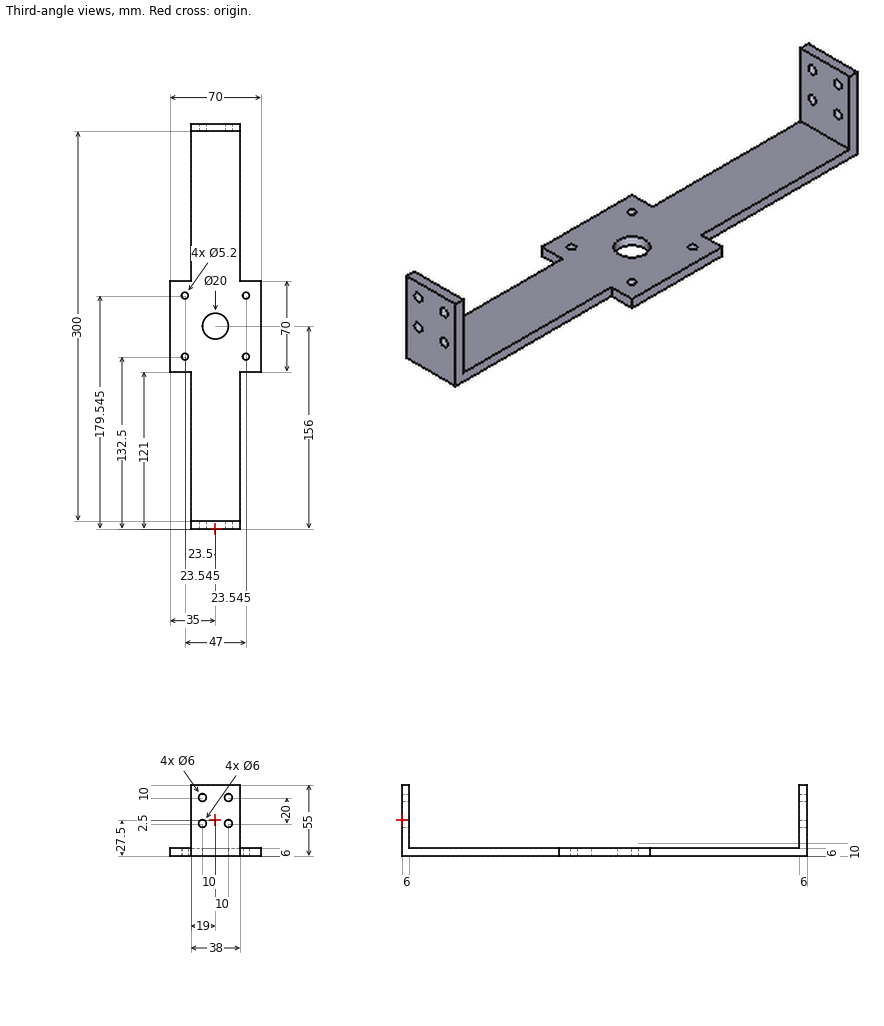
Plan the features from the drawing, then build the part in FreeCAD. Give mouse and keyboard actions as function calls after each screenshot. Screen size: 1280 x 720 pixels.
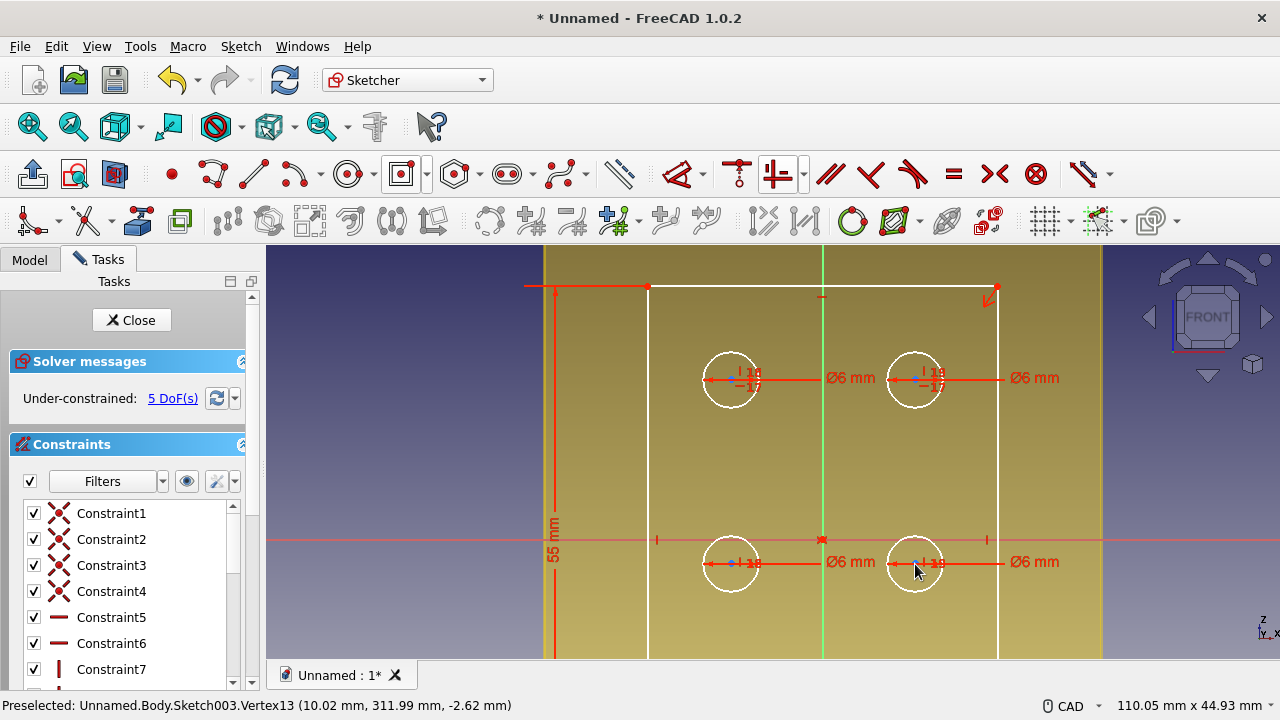
click(731, 564)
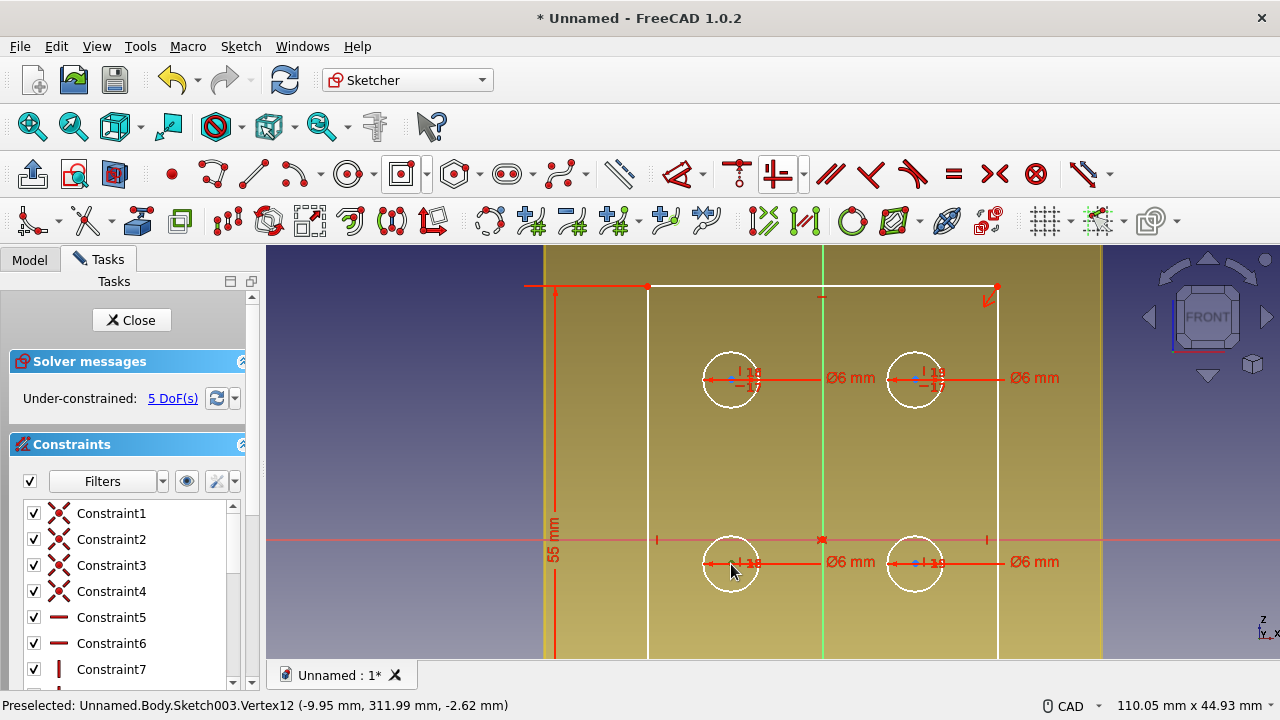
click(915, 564)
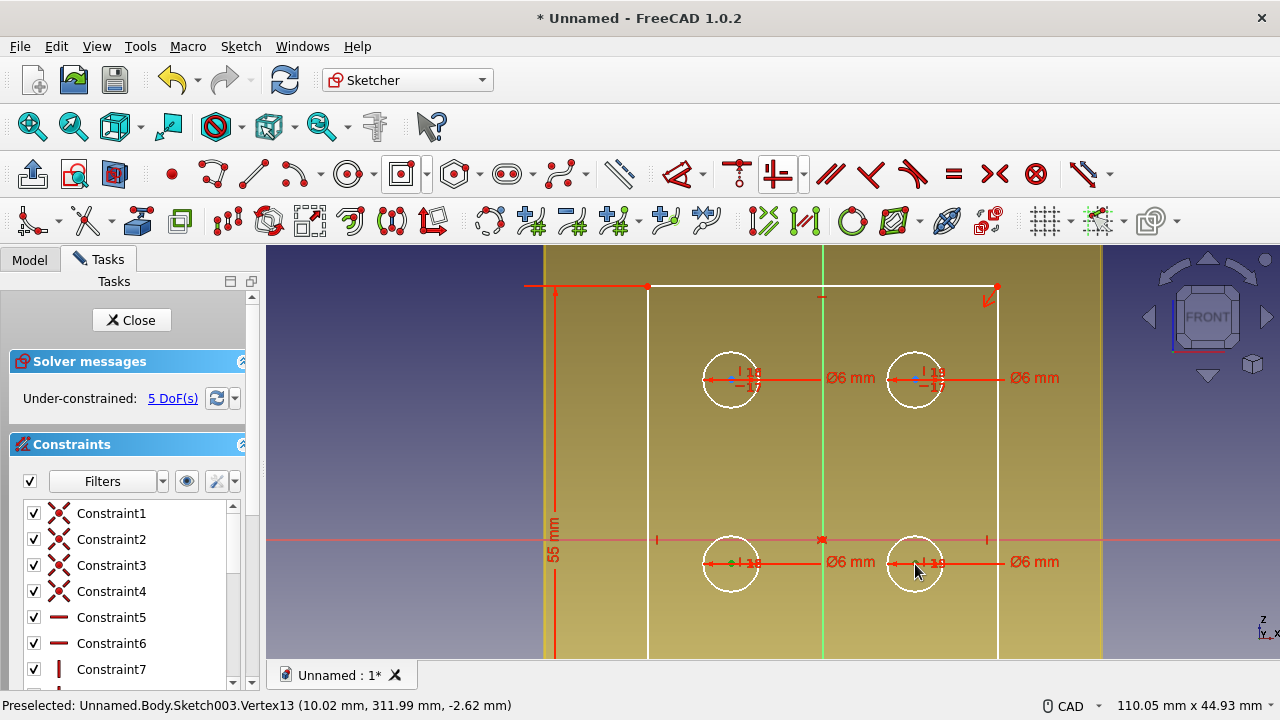
key(h)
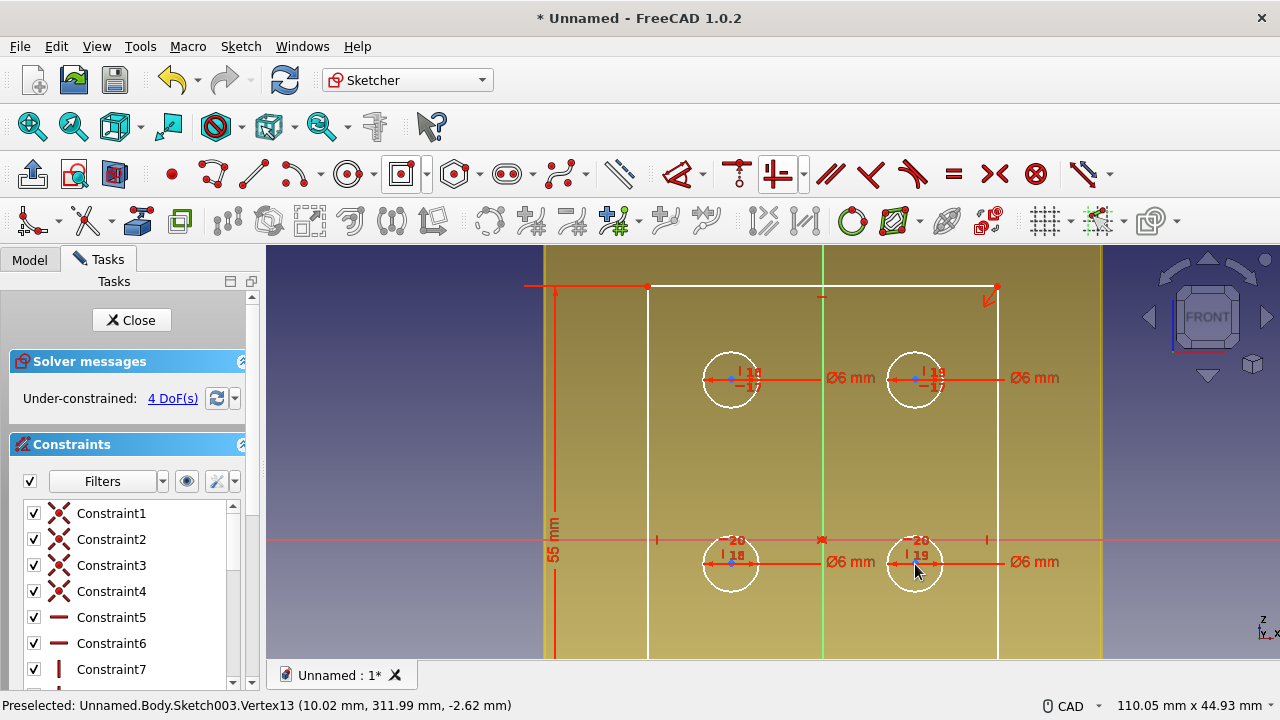
click(676, 174)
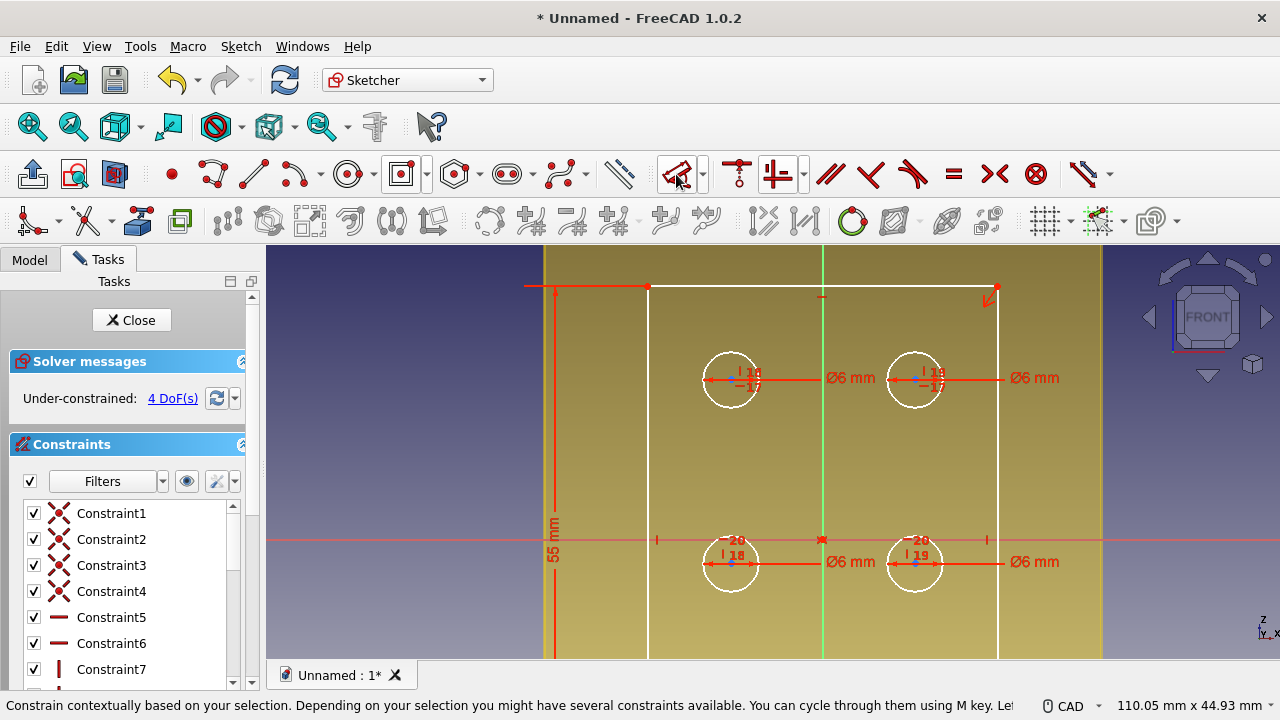
click(731, 380)
click(777, 346)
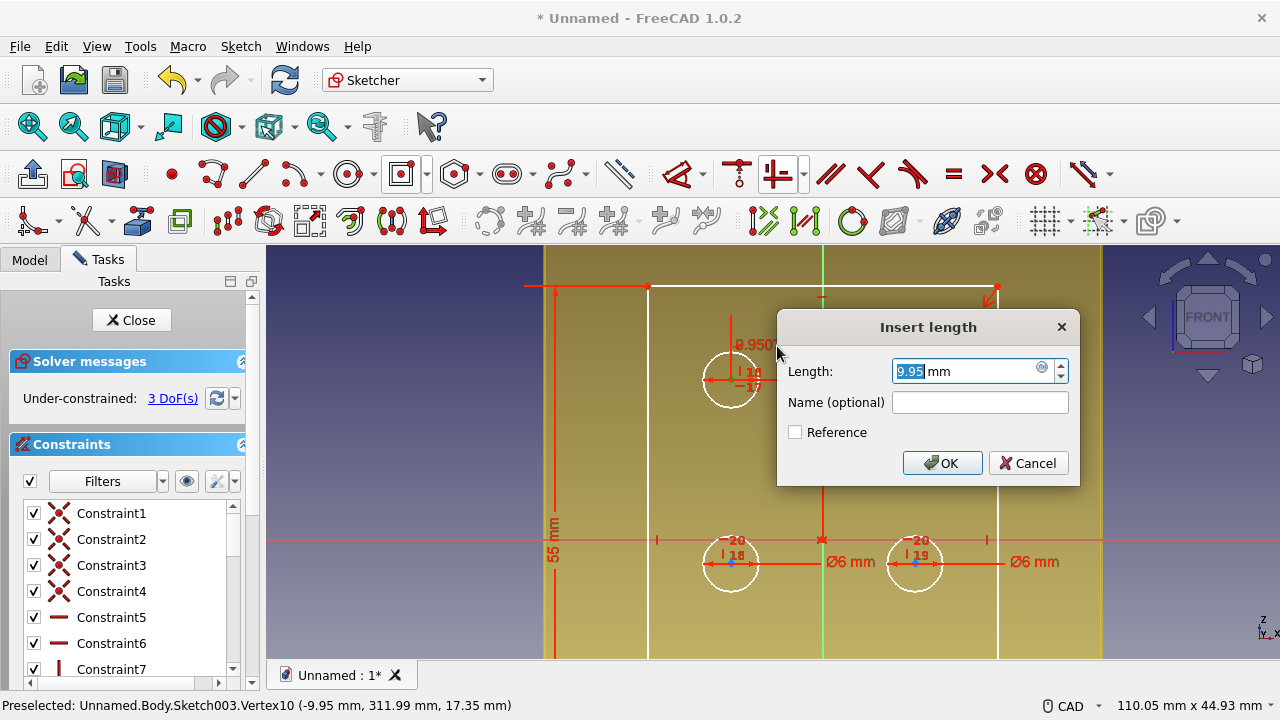
text(10)
key(Return)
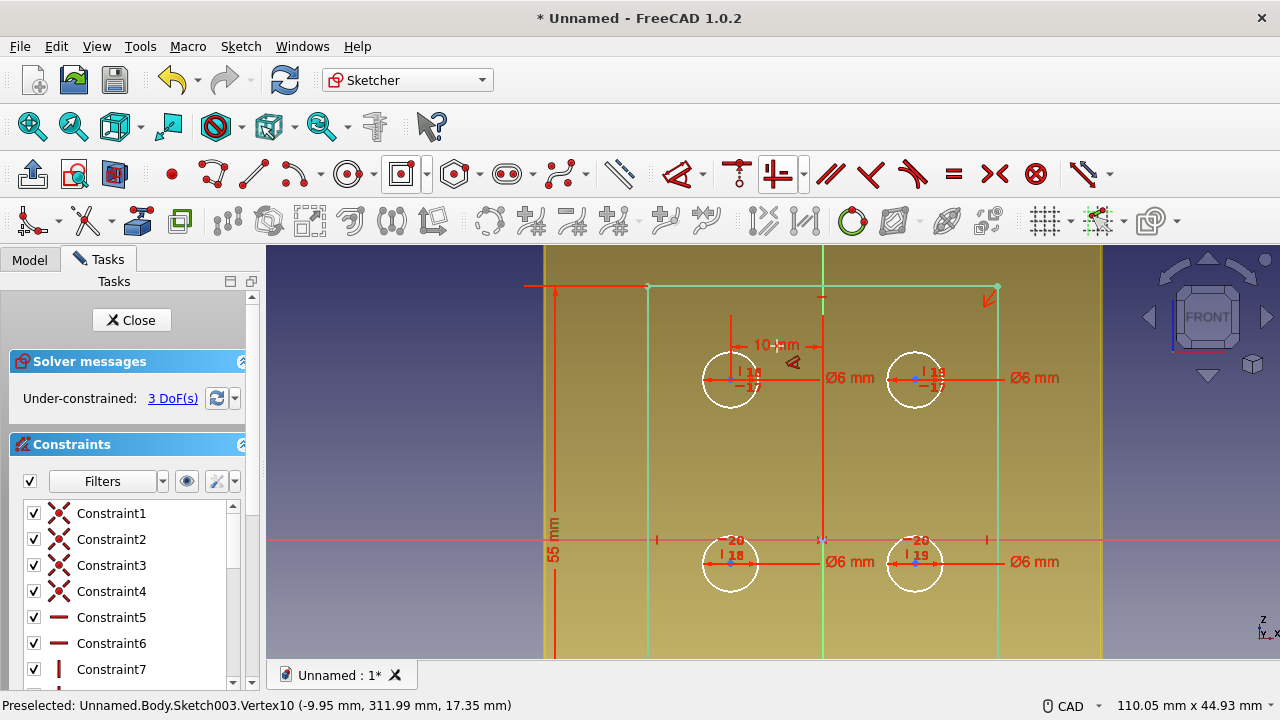
click(915, 380)
click(869, 346)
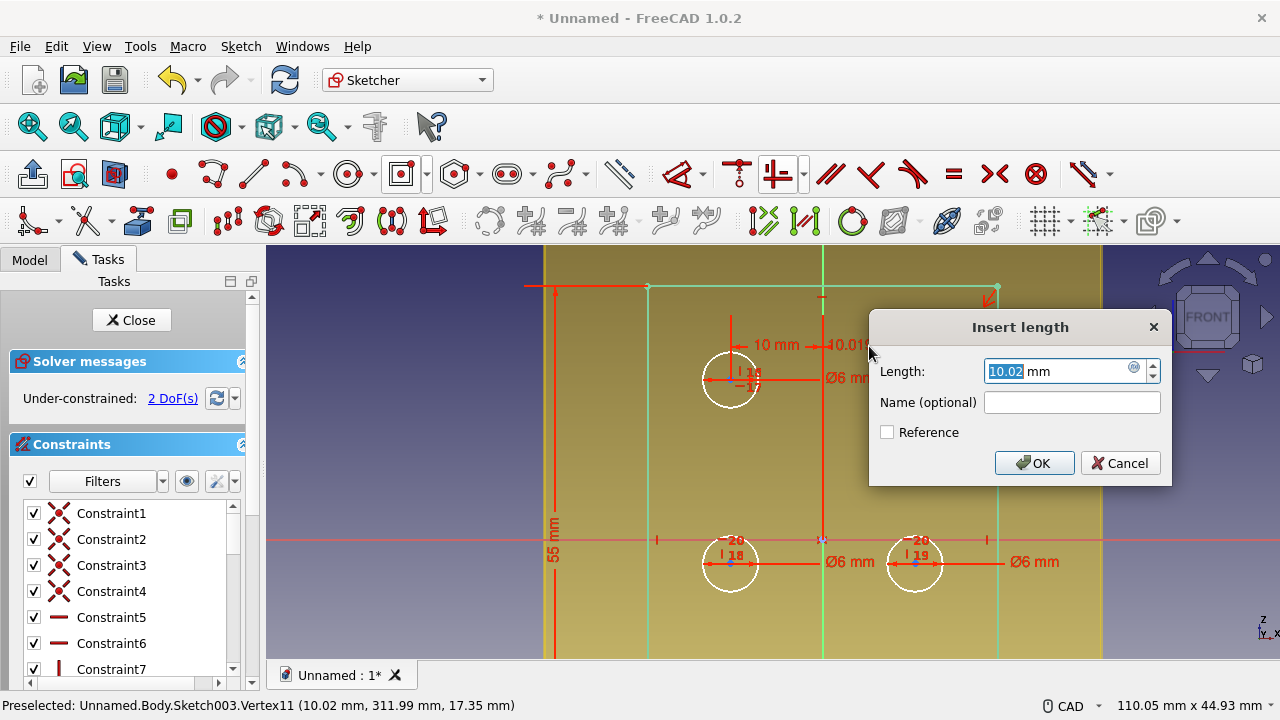
text(10)
key(Return)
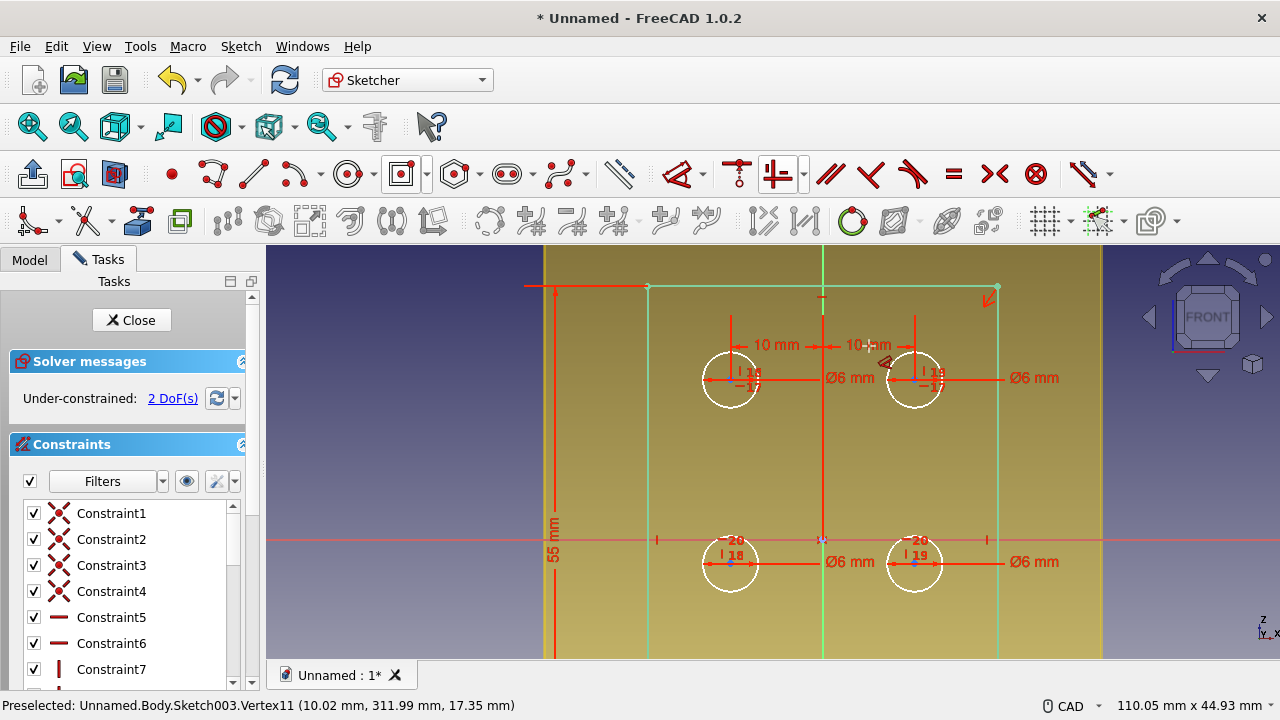
scroll(731, 564, up, 3)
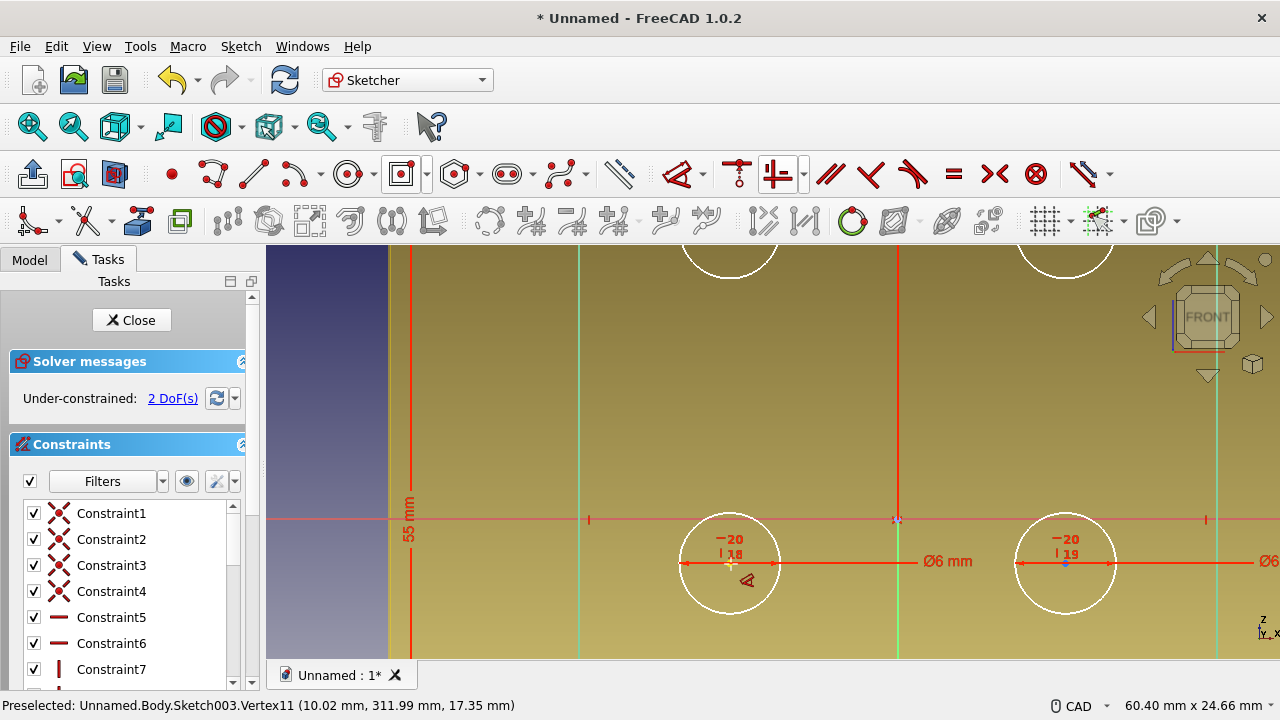
click(730, 563)
click(696, 551)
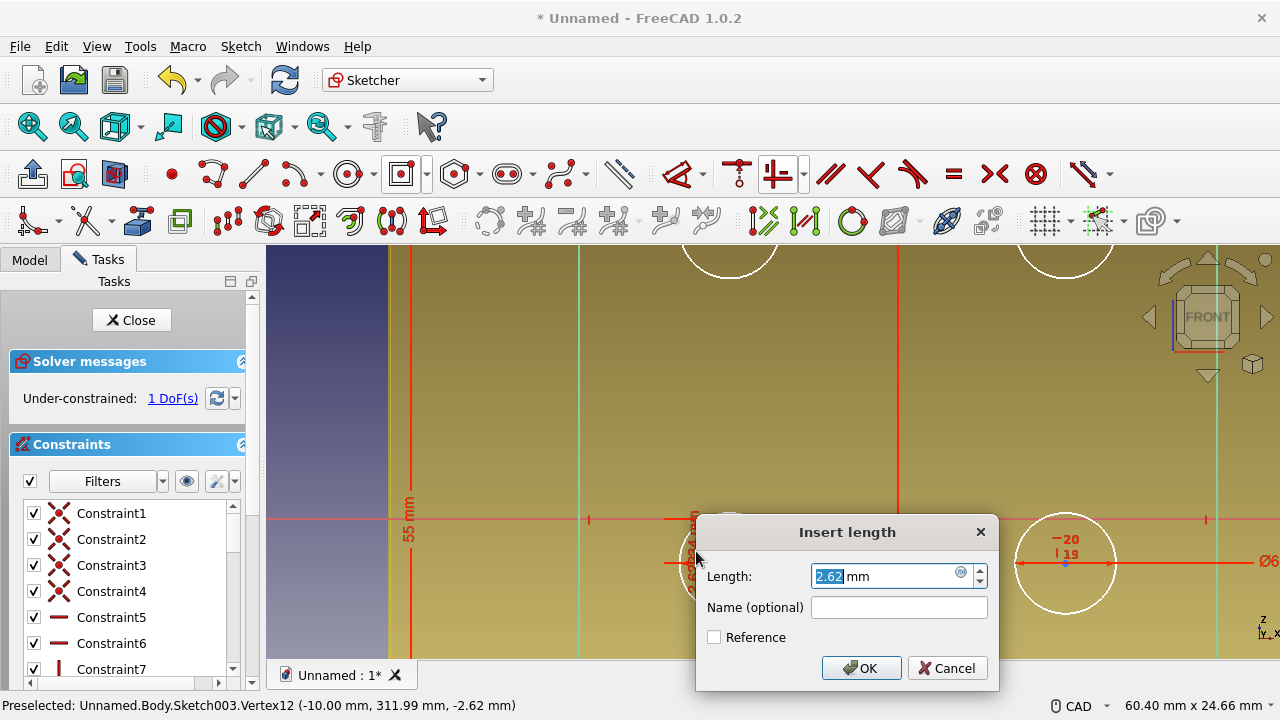
text(2.5)
key(Return)